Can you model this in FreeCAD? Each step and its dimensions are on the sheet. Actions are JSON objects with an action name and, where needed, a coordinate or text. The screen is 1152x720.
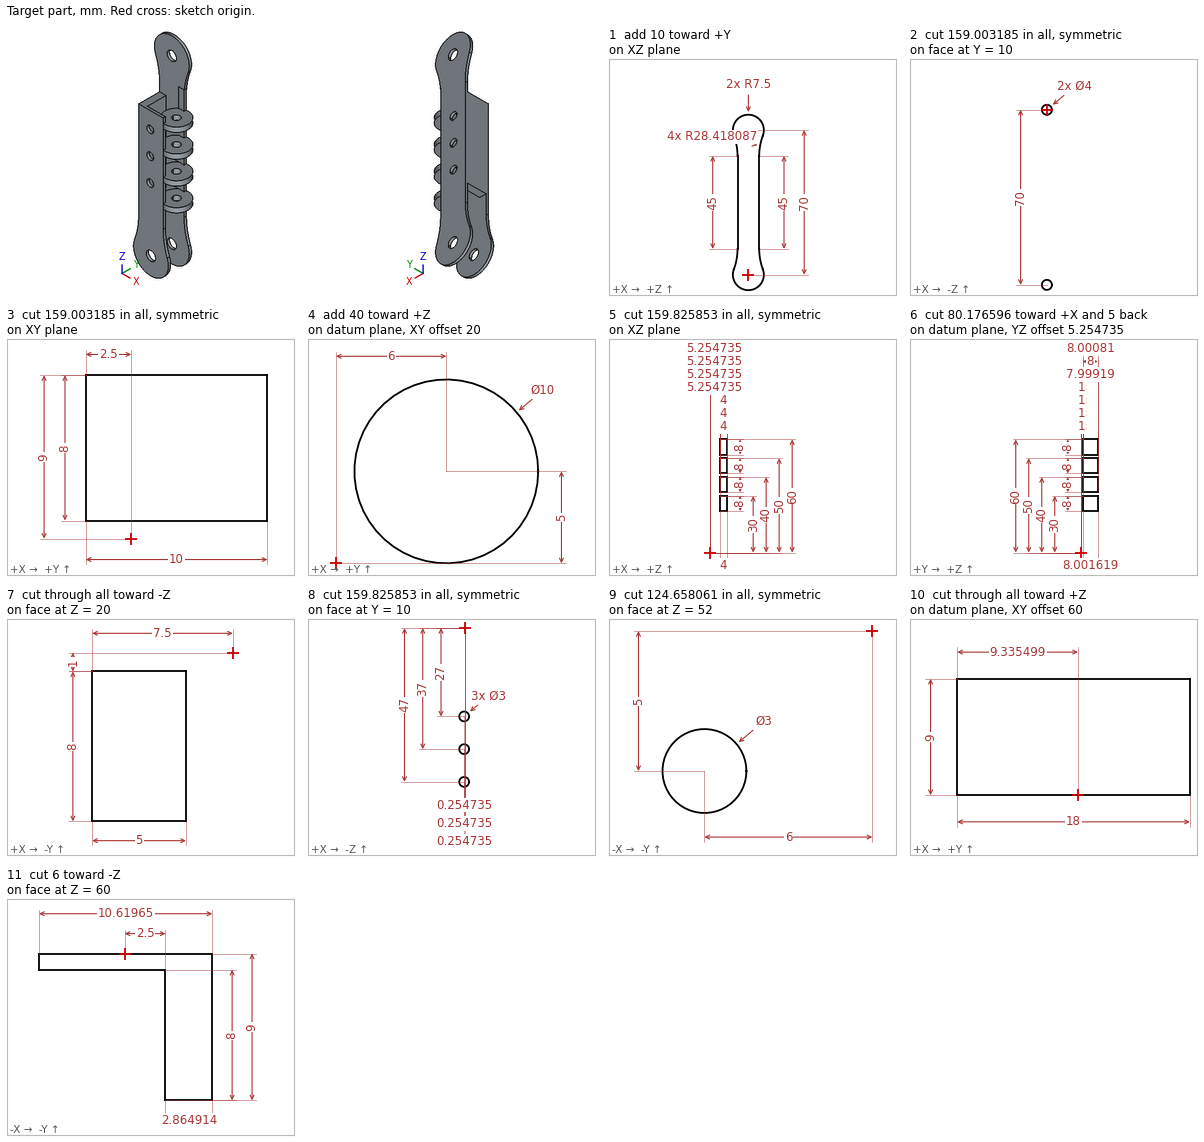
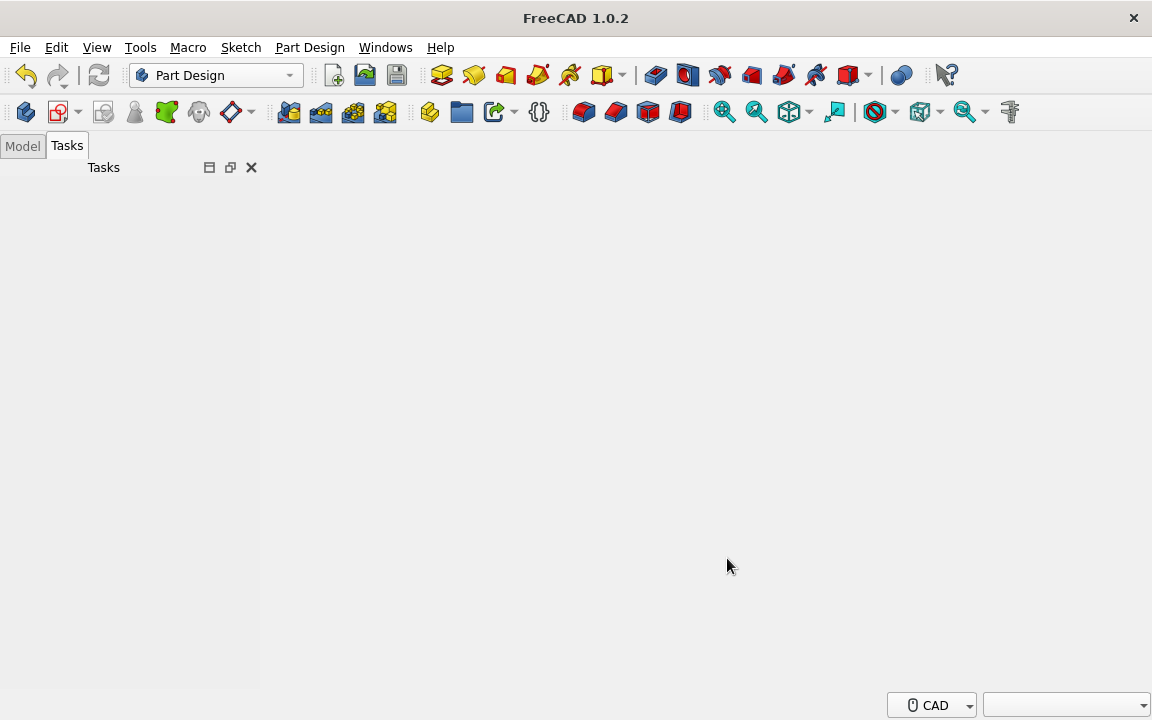
{"action": "left_click", "coordinate": [334, 76]}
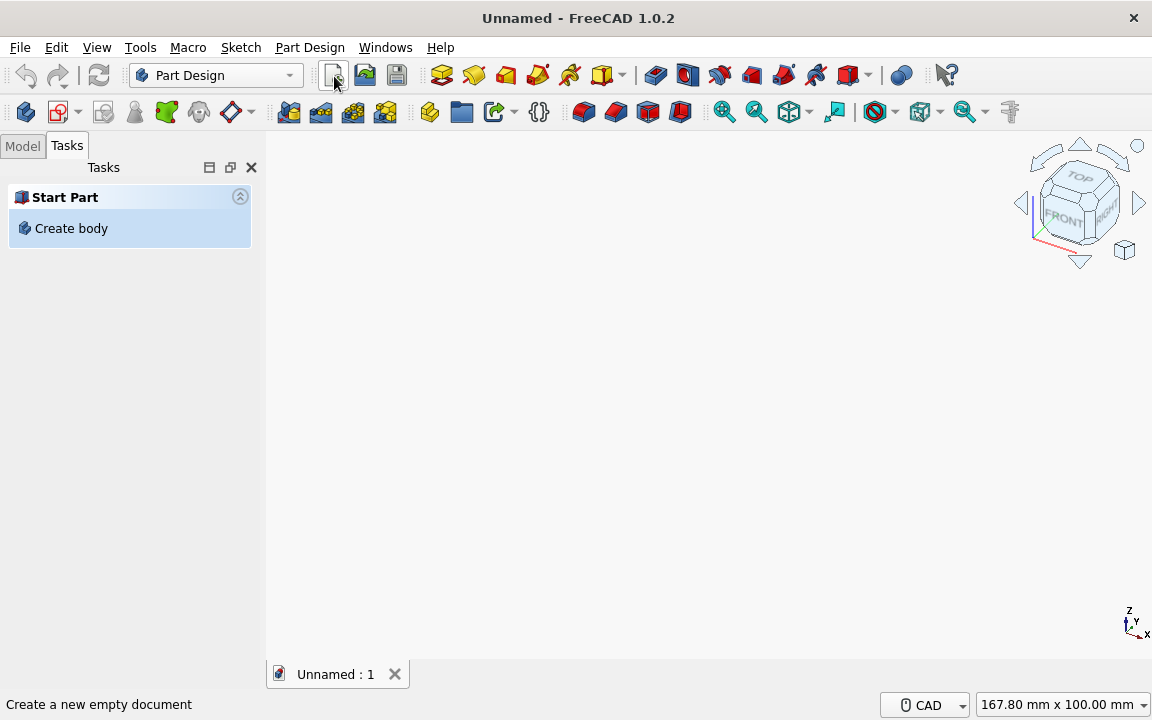
{"action": "left_click", "coordinate": [58, 112]}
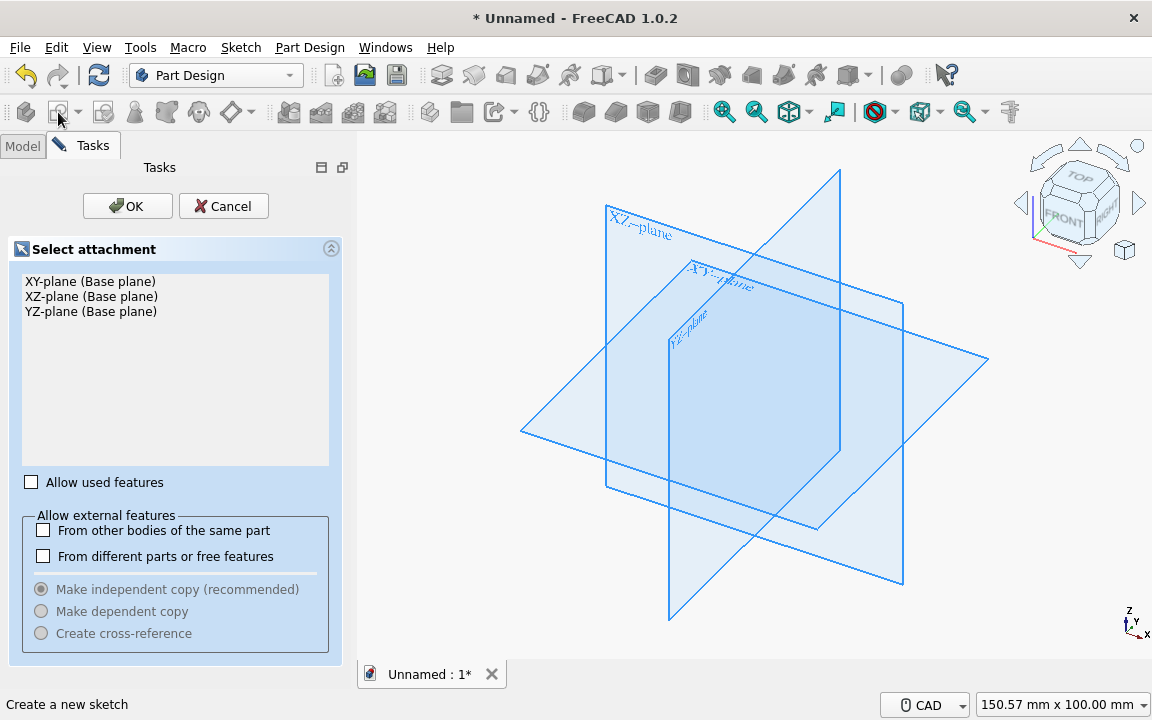
{"action": "left_click", "coordinate": [82, 296]}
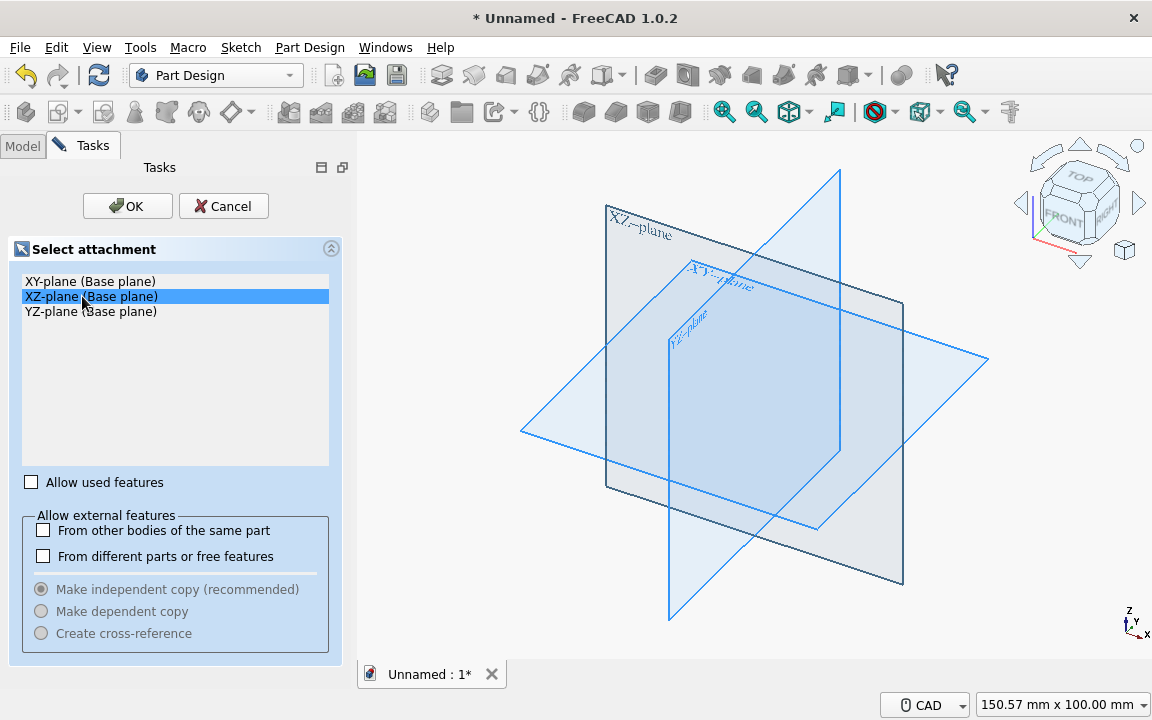
{"action": "left_click", "coordinate": [128, 206]}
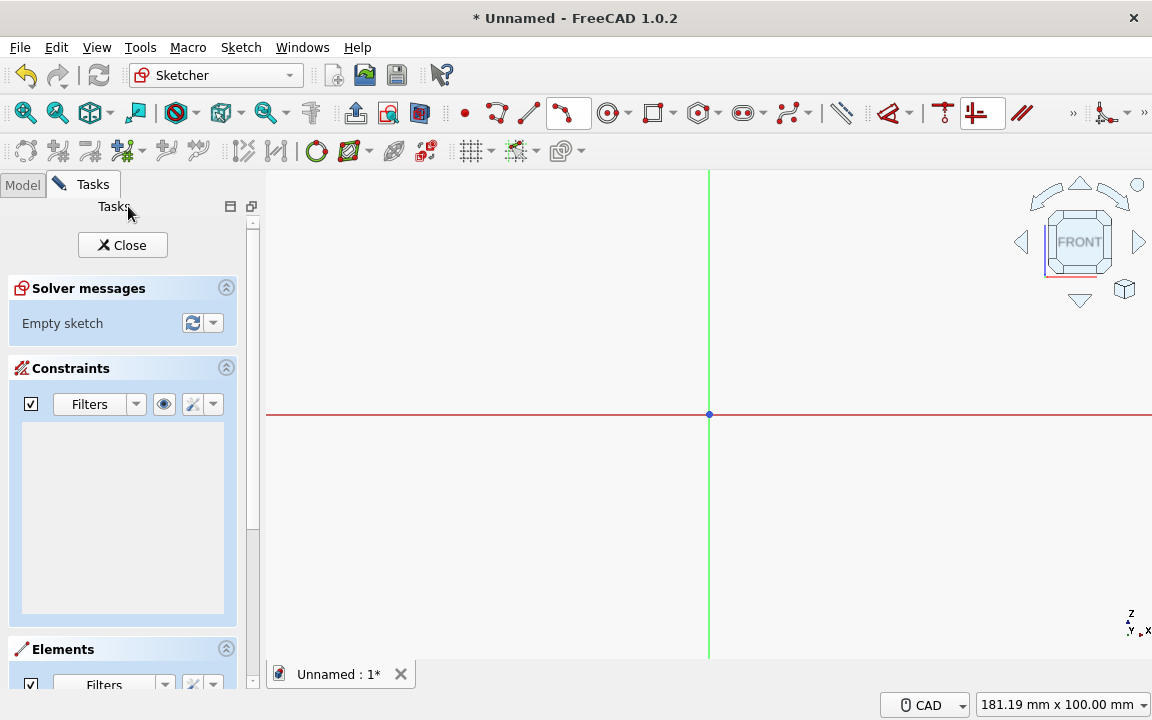
{"action": "scroll", "coordinate": [501, 631], "scroll_direction": "down", "scroll_amount": 2}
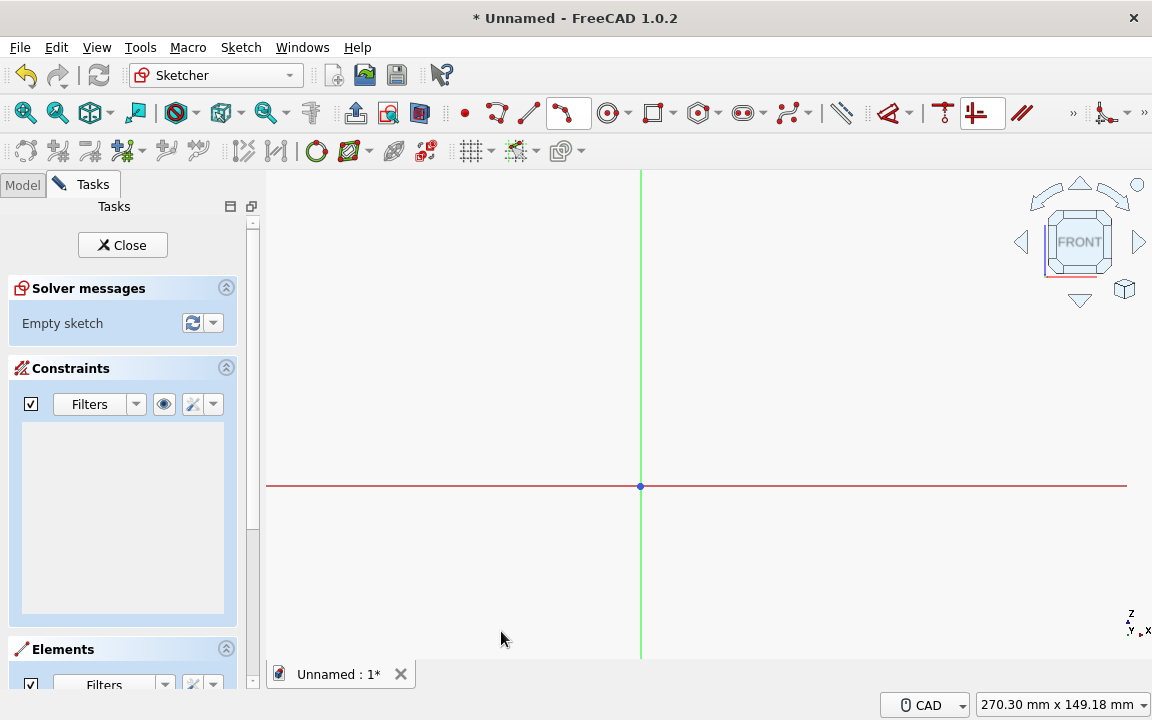
{"action": "left_click", "coordinate": [530, 114]}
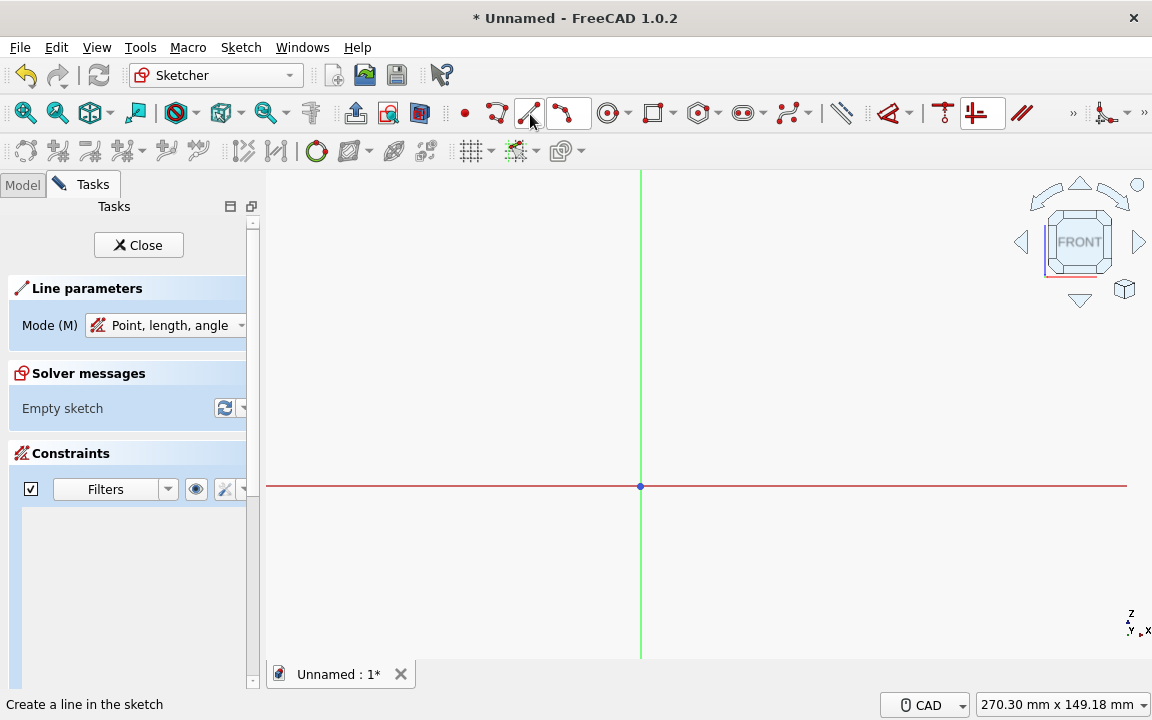
{"action": "left_click", "coordinate": [623, 445]}
{"action": "left_click", "coordinate": [623, 298]}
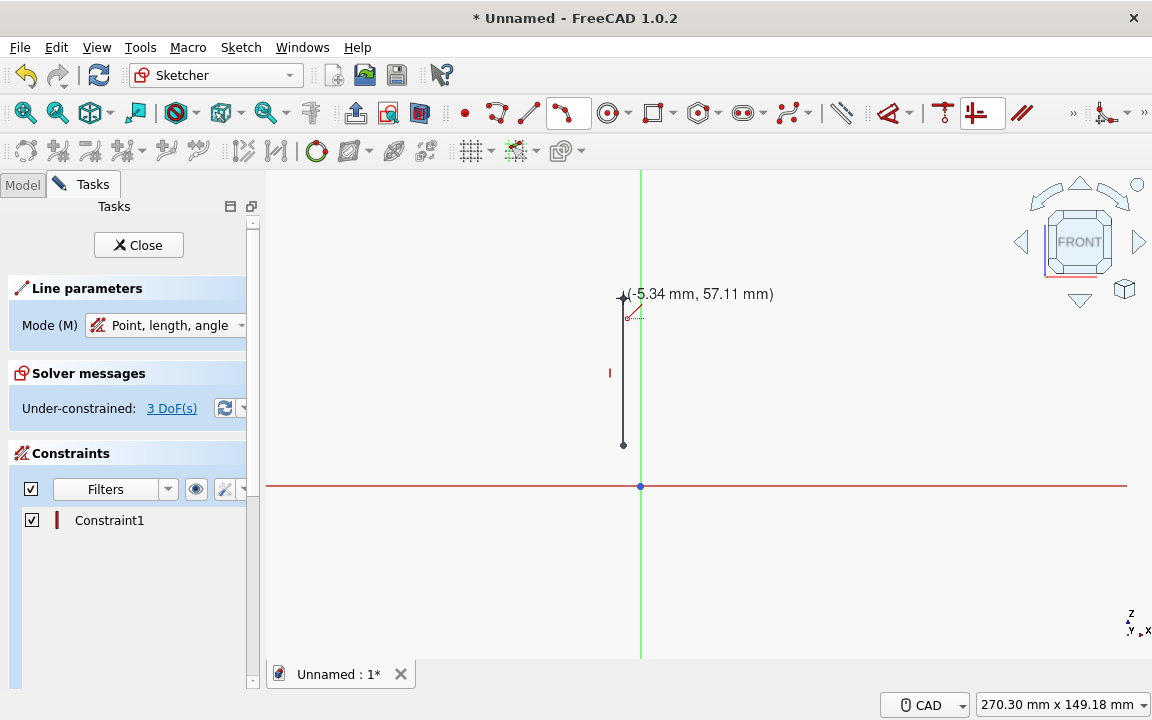
{"action": "left_click", "coordinate": [658, 298]}
{"action": "left_click", "coordinate": [658, 445]}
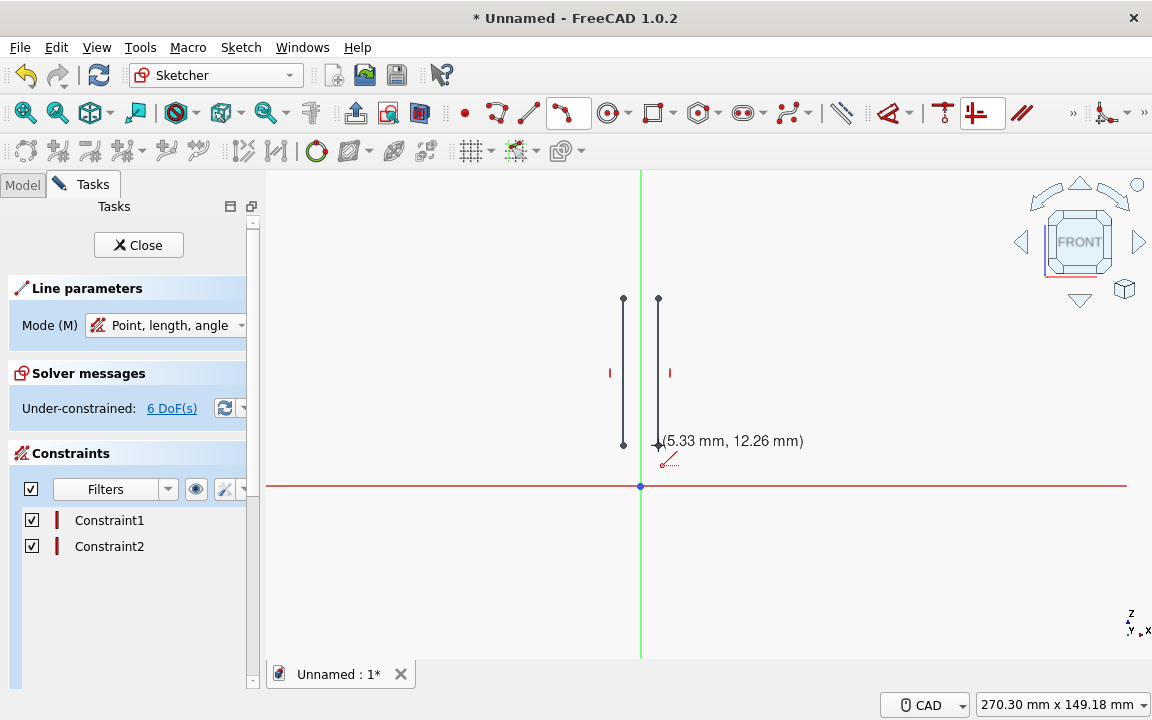
{"action": "left_click", "coordinate": [562, 114]}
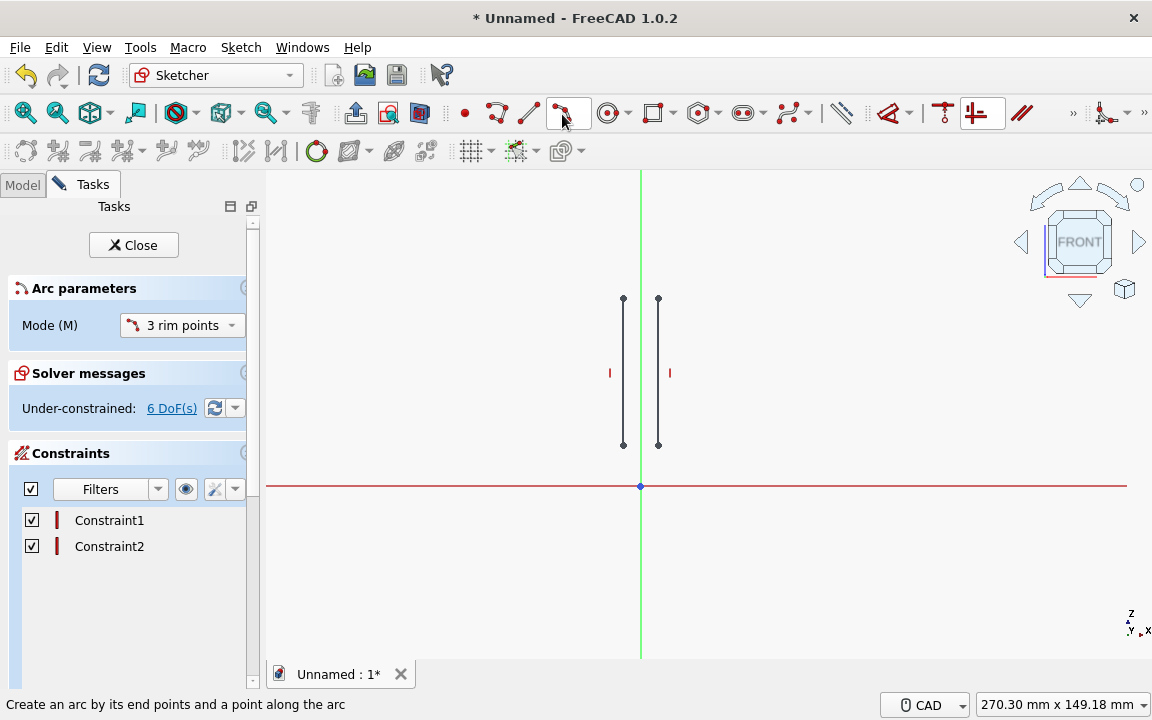
{"action": "left_click", "coordinate": [623, 299]}
{"action": "left_click", "coordinate": [617, 265]}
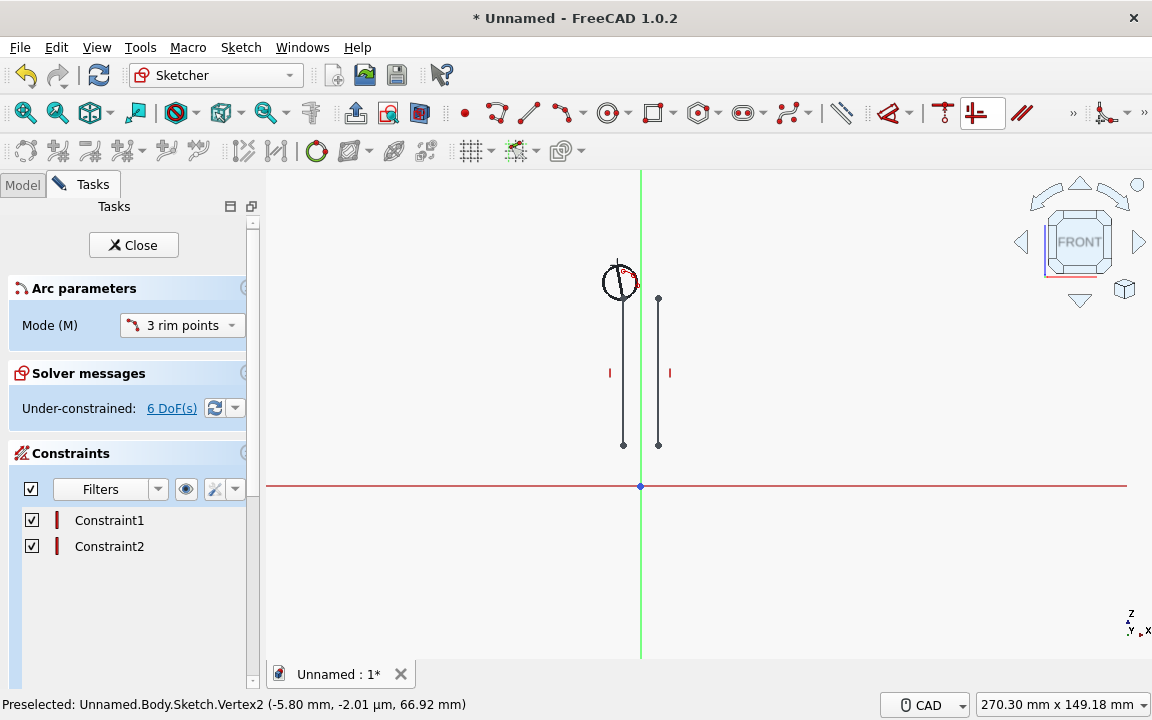
{"action": "scroll", "coordinate": [622, 281], "scroll_direction": "up", "scroll_amount": 12}